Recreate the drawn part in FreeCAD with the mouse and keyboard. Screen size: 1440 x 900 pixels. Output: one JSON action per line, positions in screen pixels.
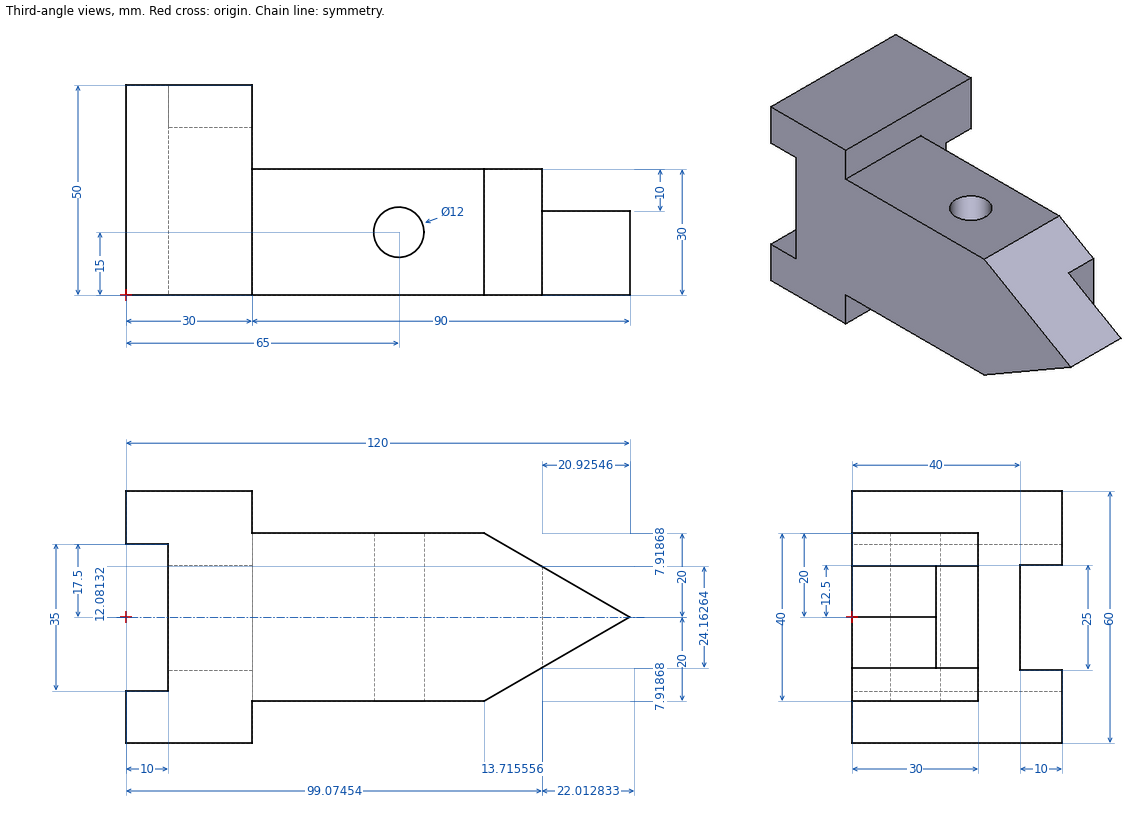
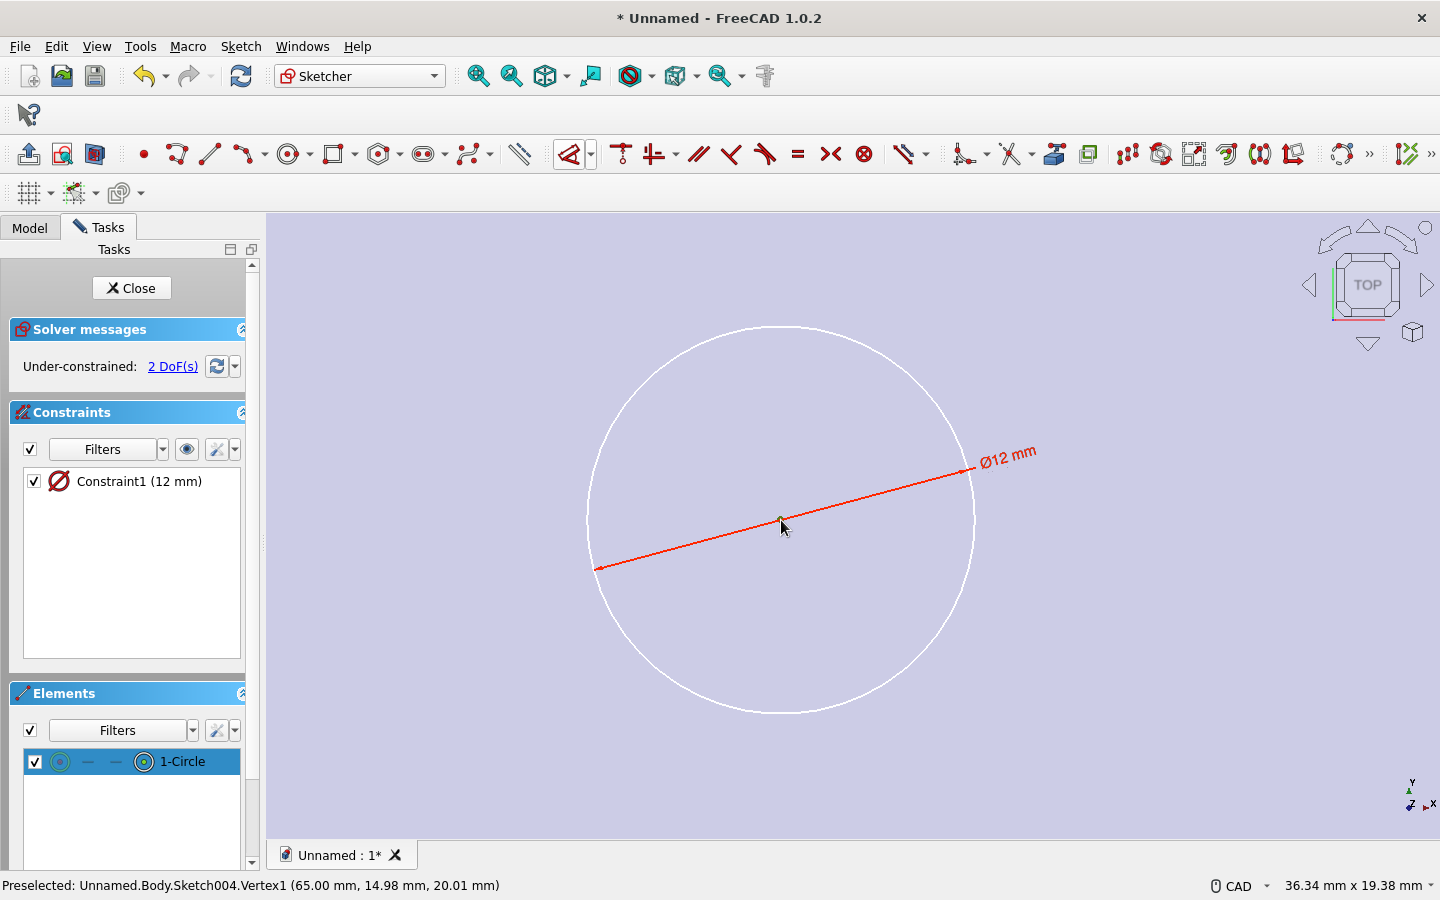
{"action": "key", "text": "l"}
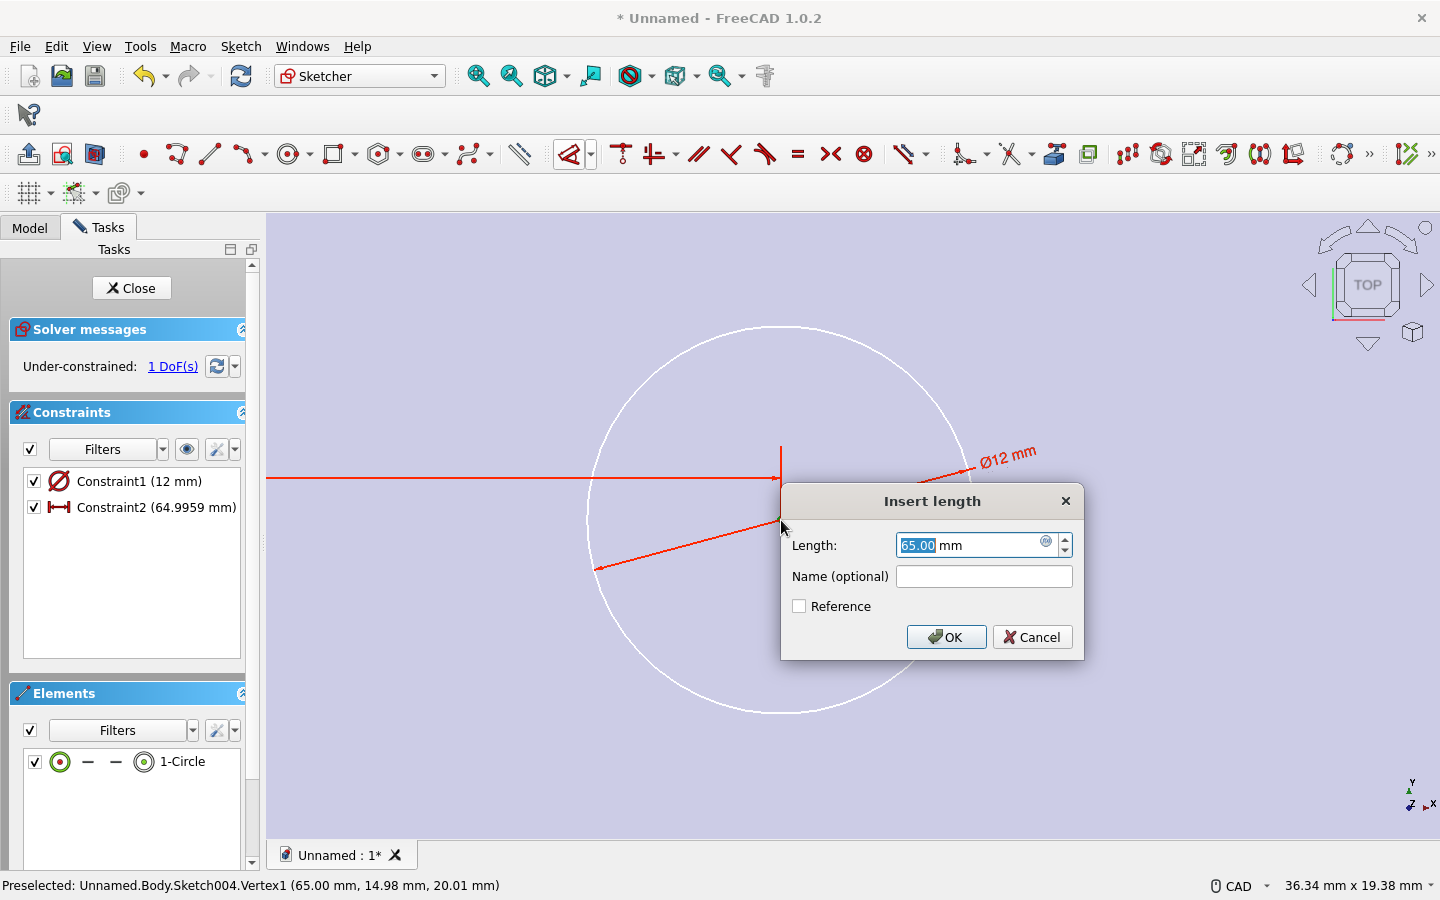
{"action": "type", "text": "65"}
{"action": "key", "text": "Return"}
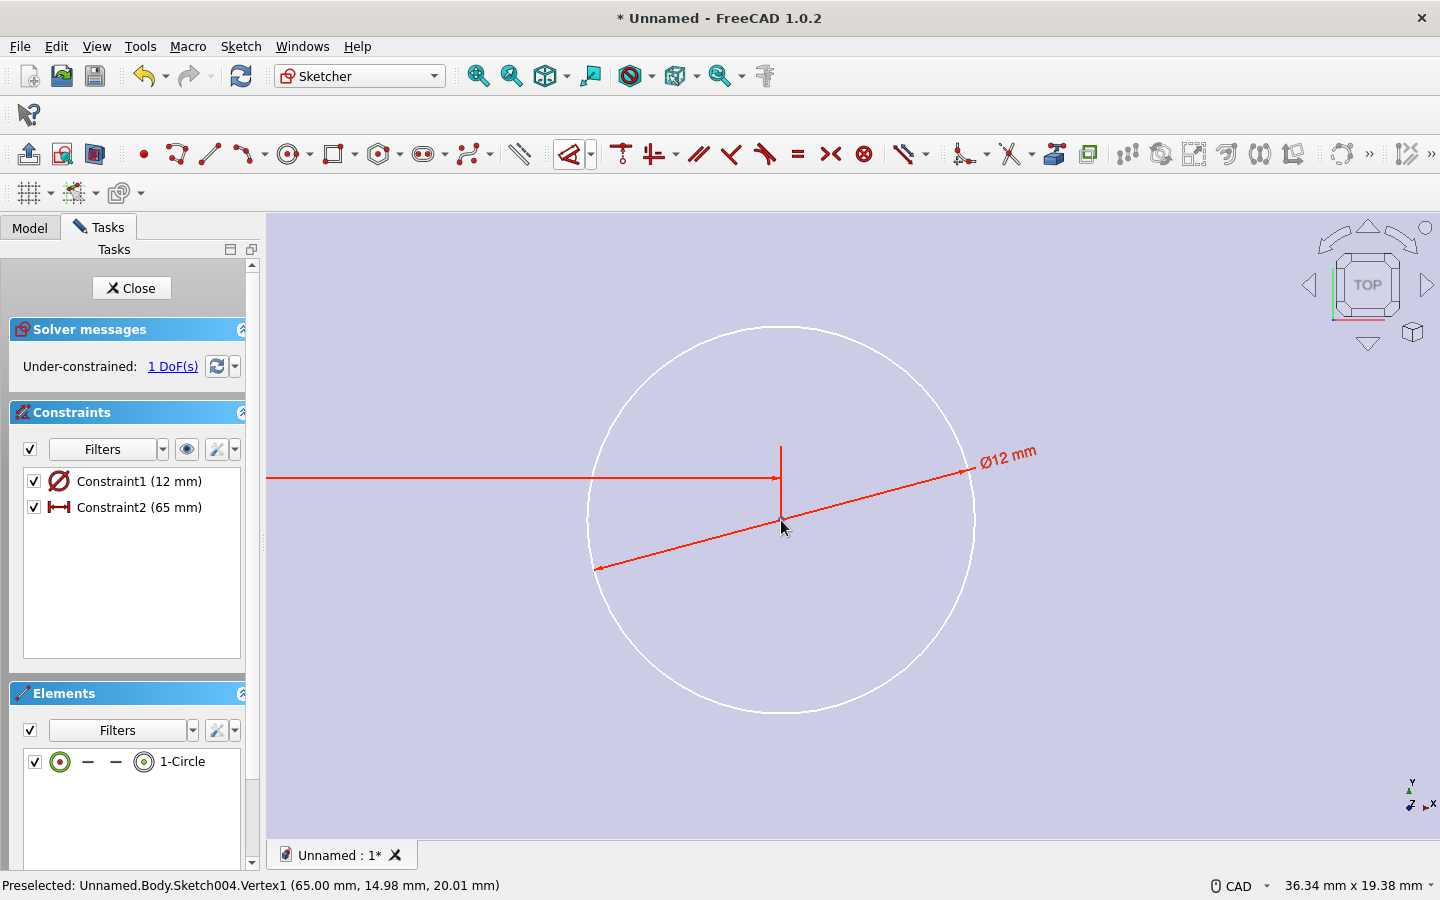
{"action": "left_click", "coordinate": [781, 520]}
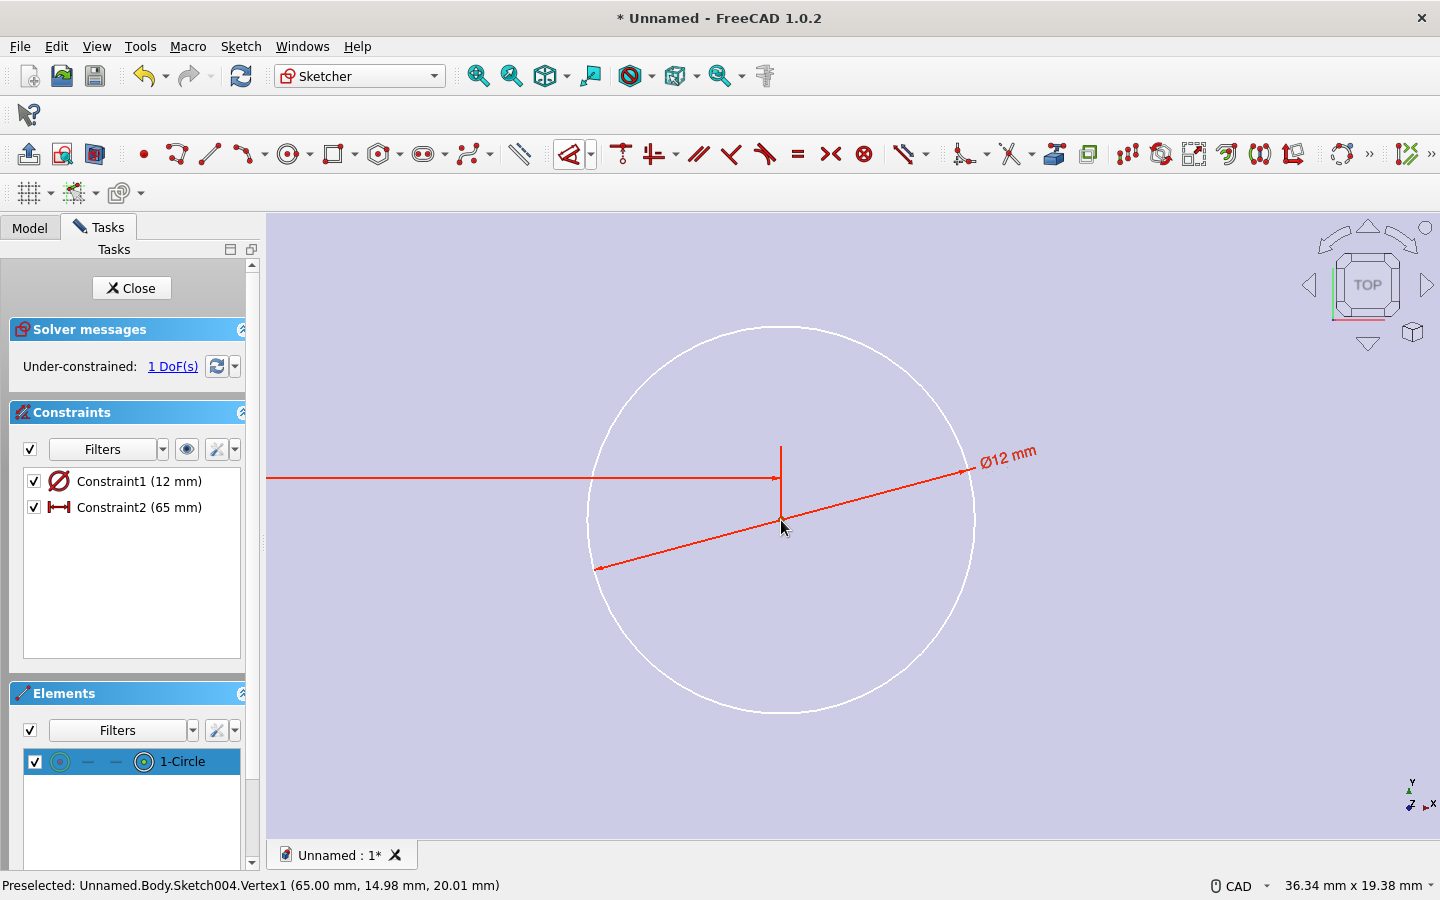
{"action": "key", "text": "i"}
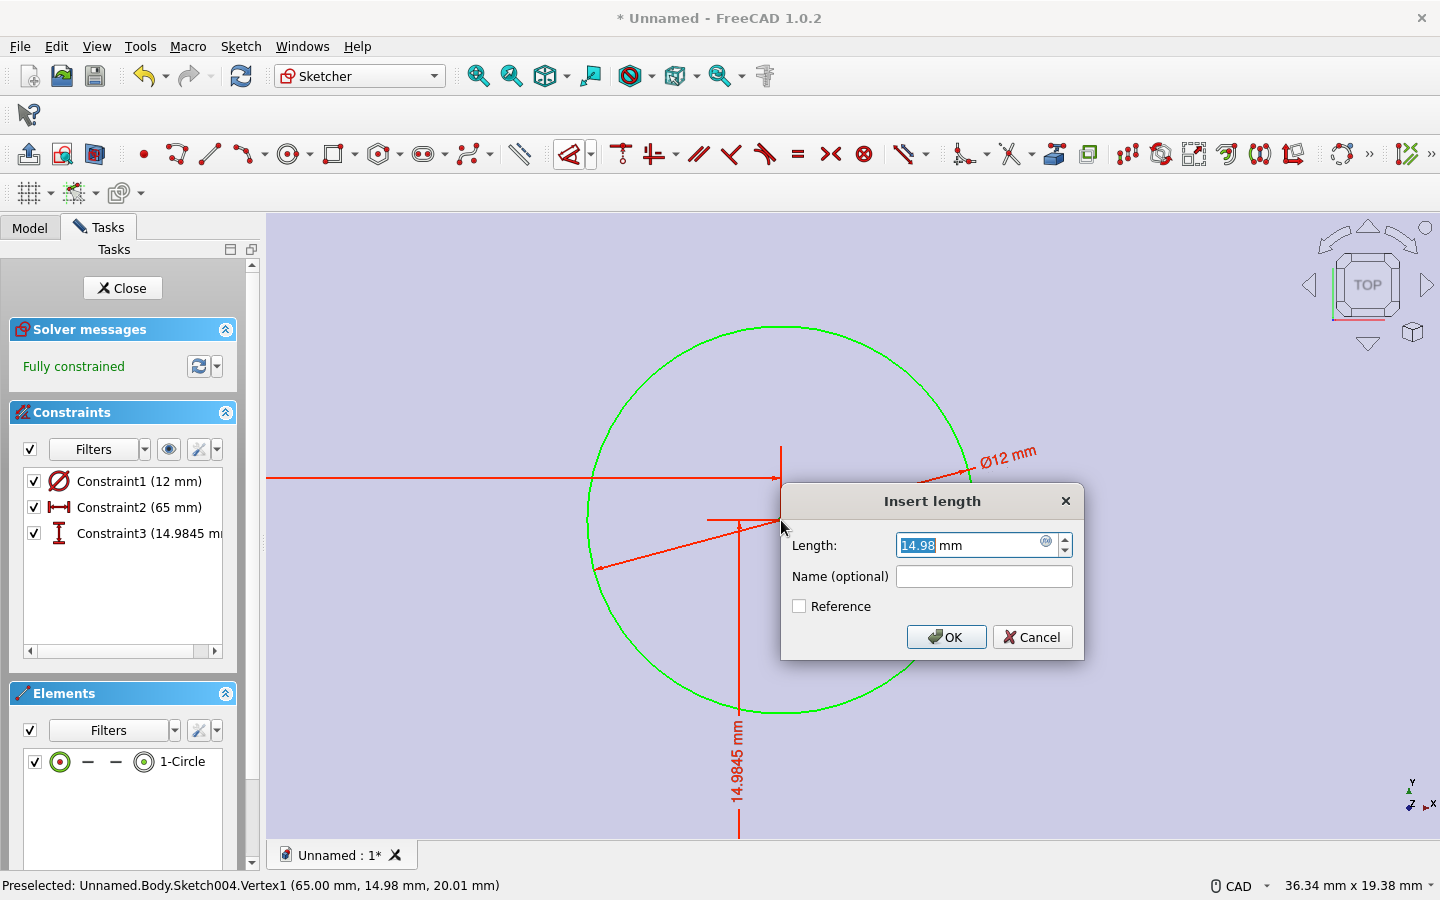
{"action": "type", "text": "15"}
{"action": "key", "text": "Return"}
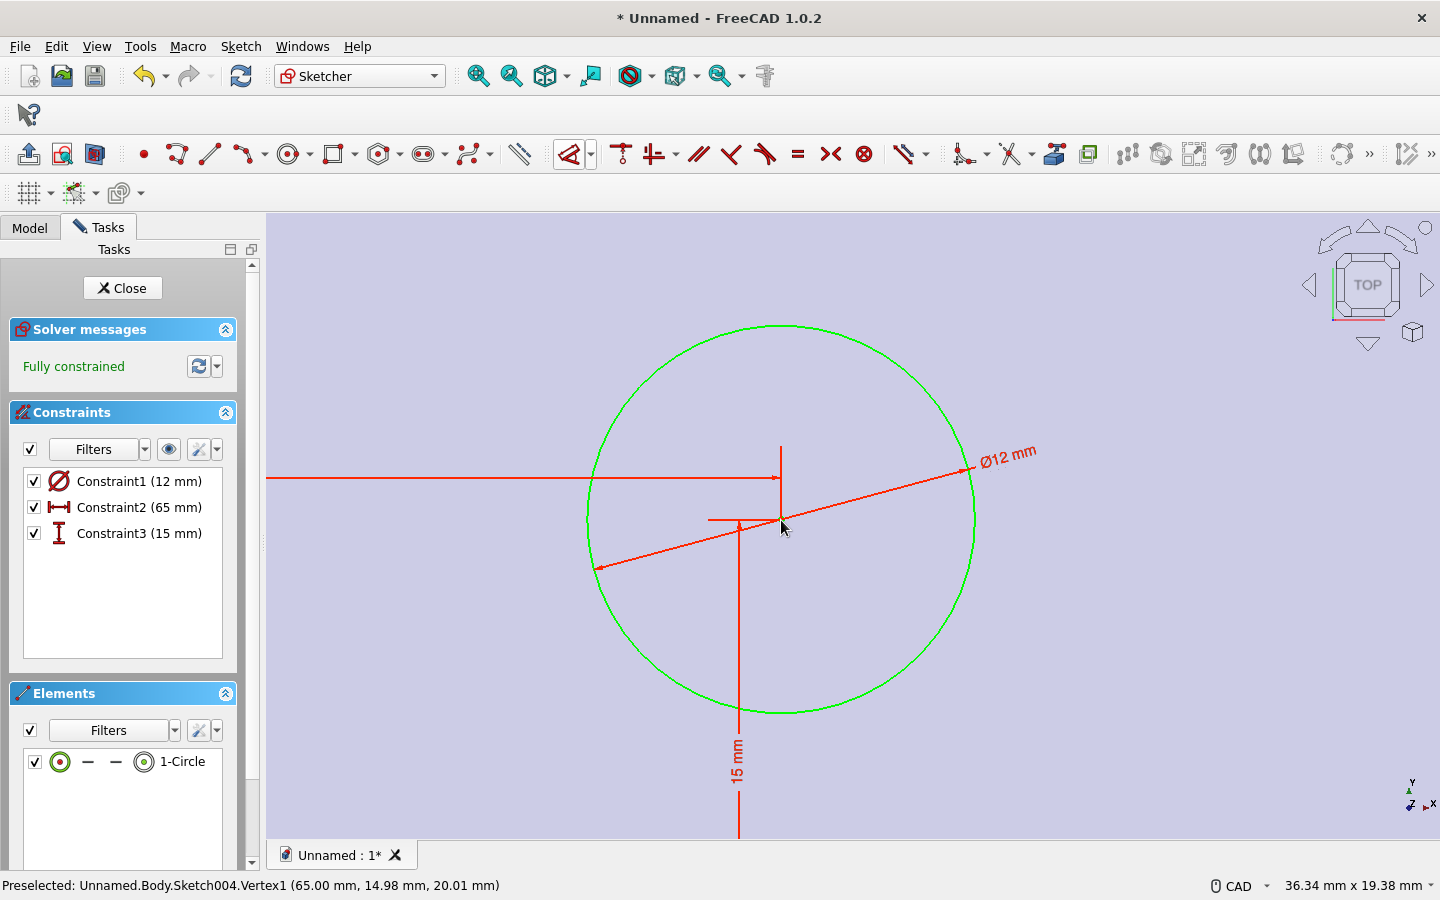
{"action": "left_click", "coordinate": [123, 288]}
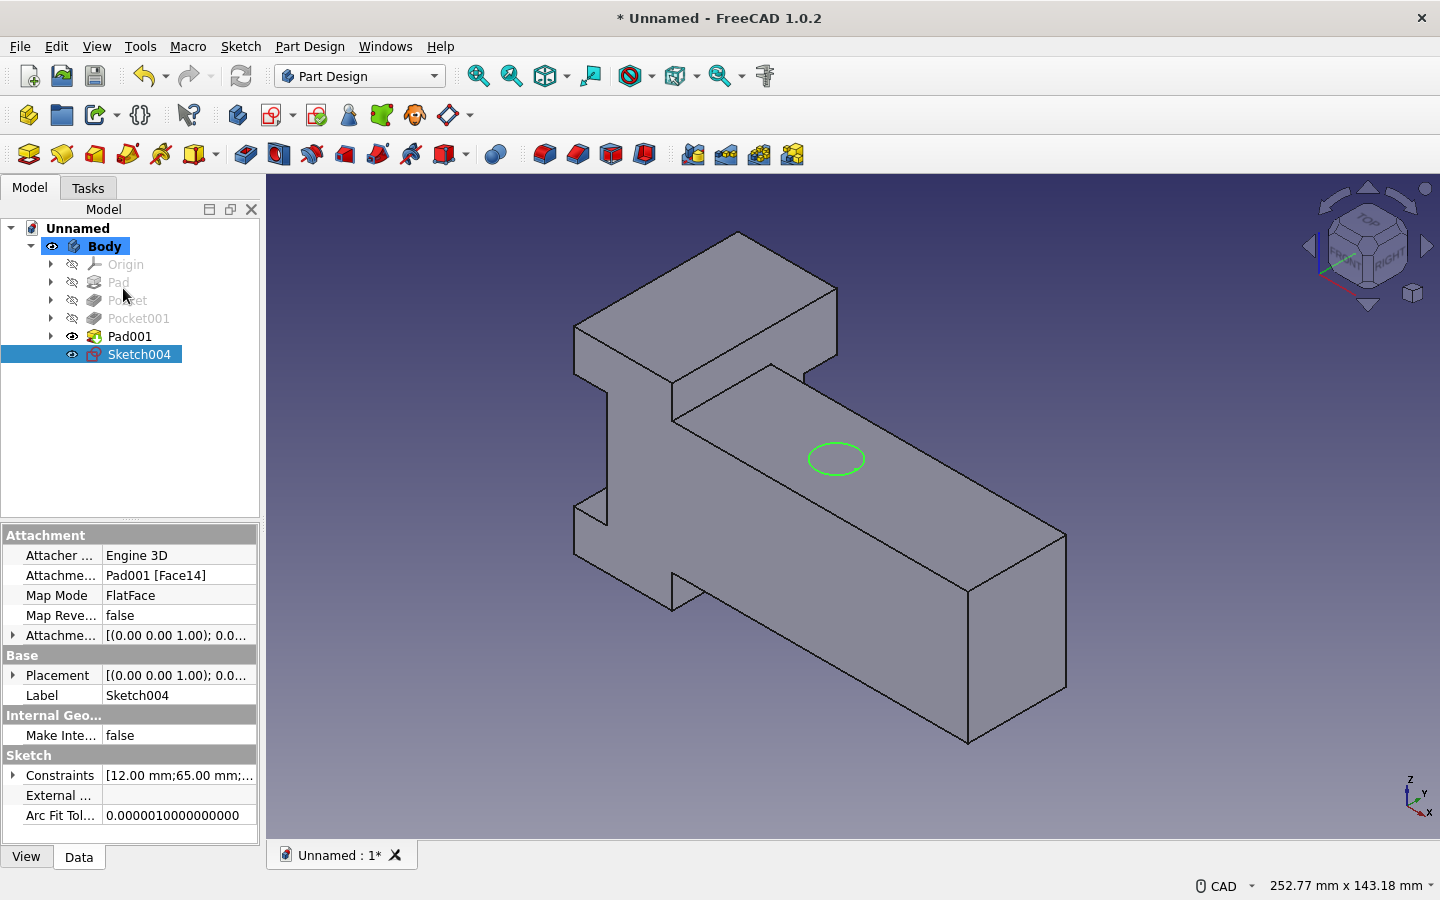
{"action": "left_click", "coordinate": [246, 154]}